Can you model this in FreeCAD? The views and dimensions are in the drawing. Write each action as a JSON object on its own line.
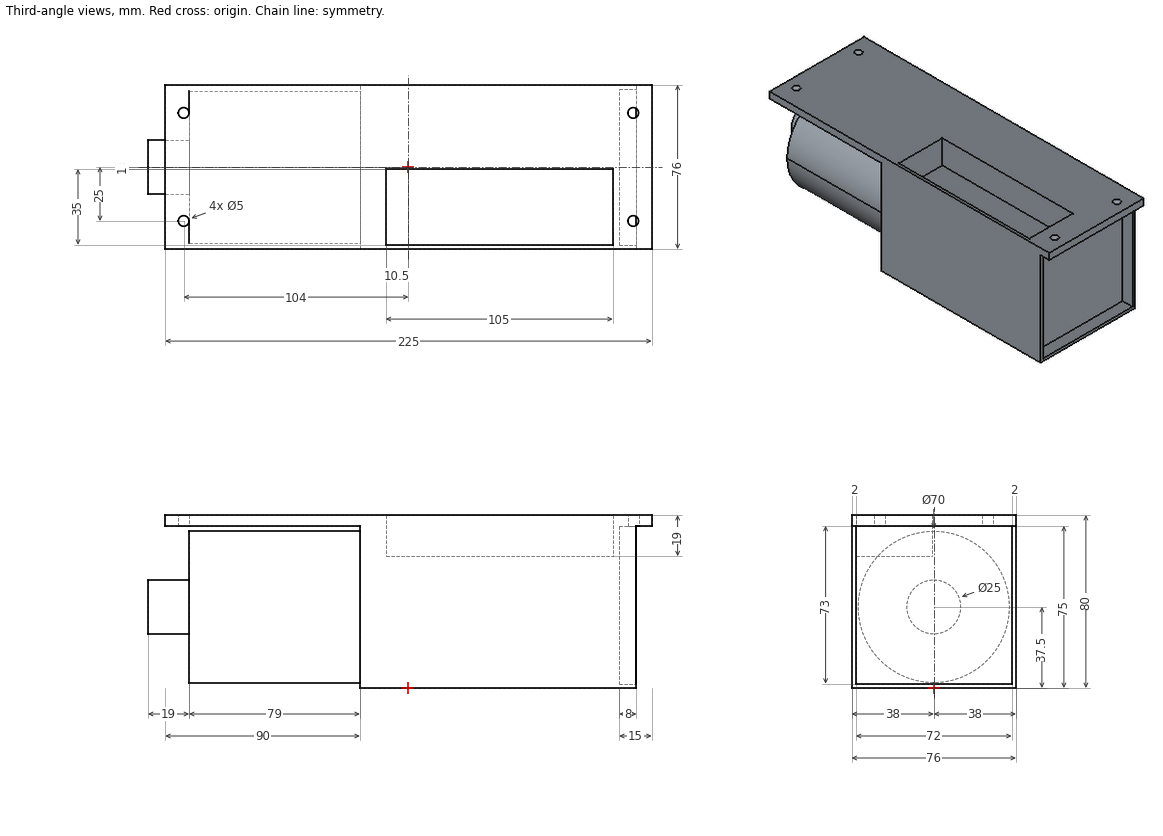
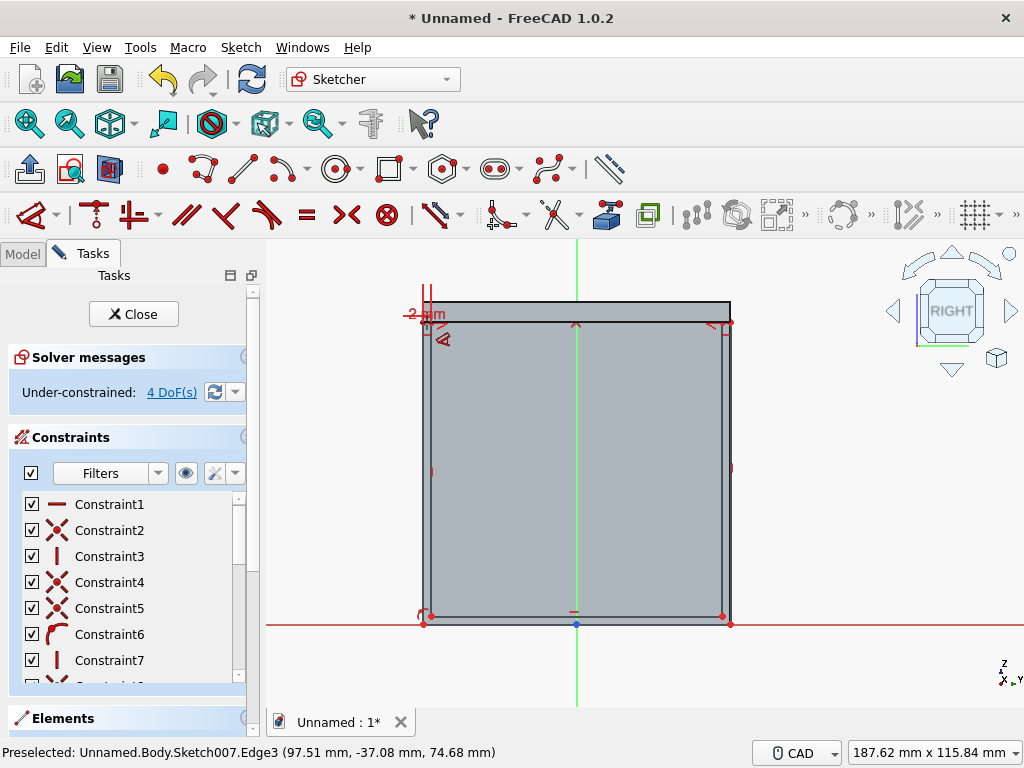
{"action": "scroll", "coordinate": [728, 323], "scroll_direction": "up", "scroll_amount": 9}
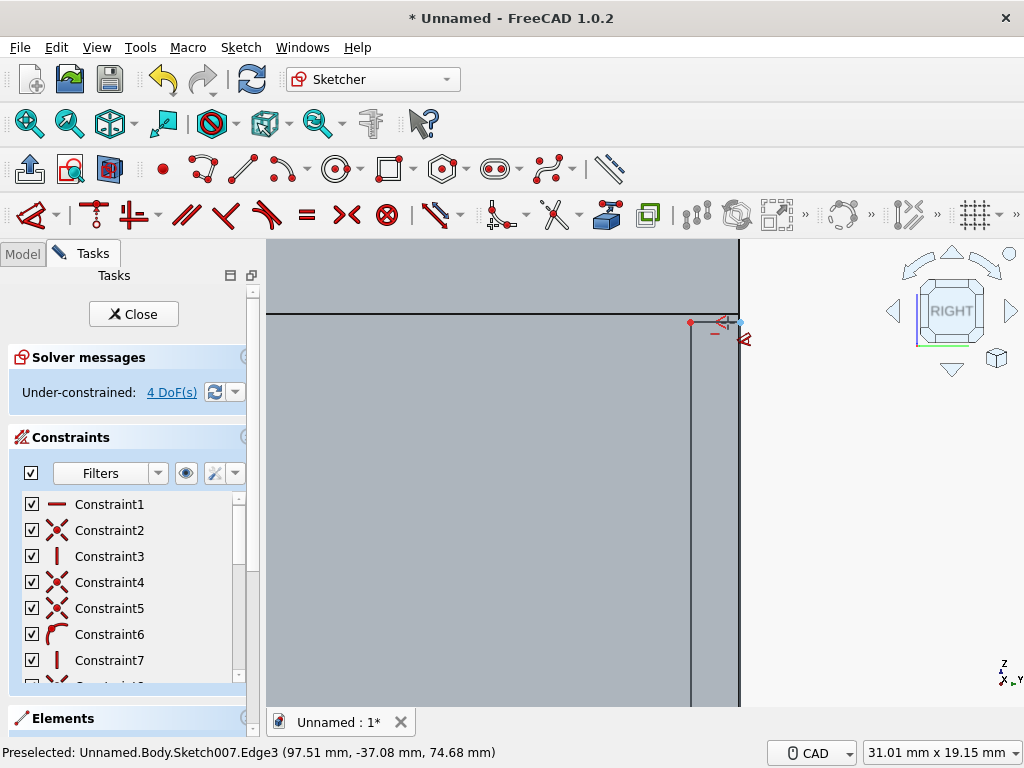
{"action": "left_click", "coordinate": [725, 322]}
{"action": "left_click", "coordinate": [715, 288]}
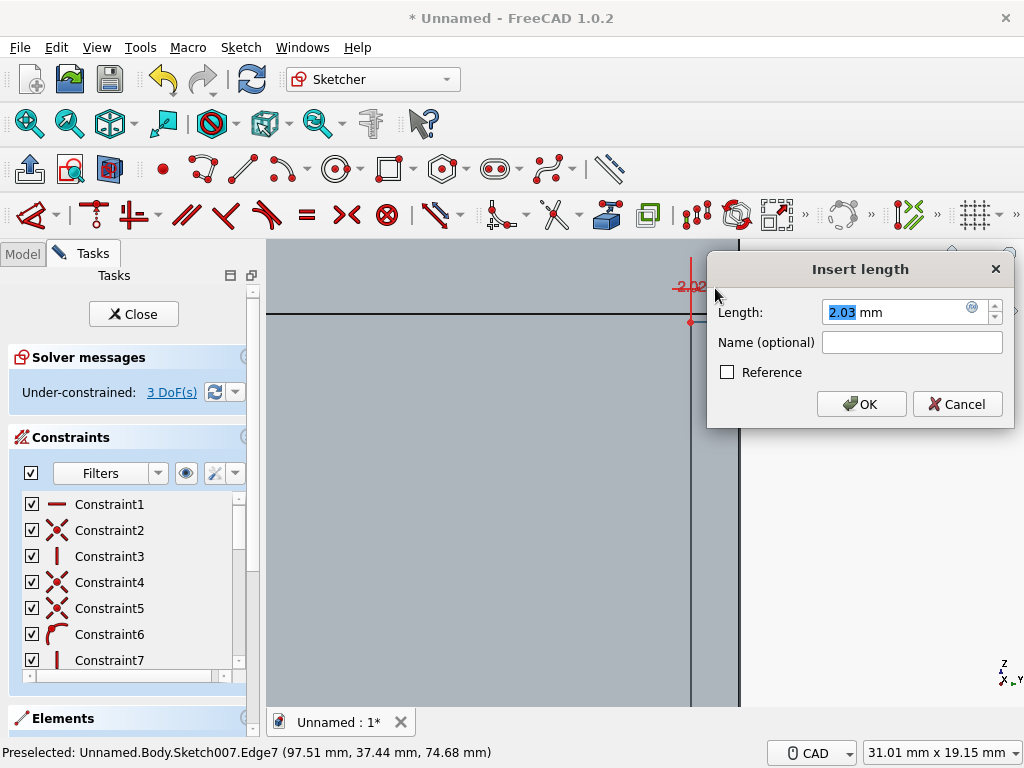
{"action": "type", "text": "2"}
{"action": "key", "text": "Return"}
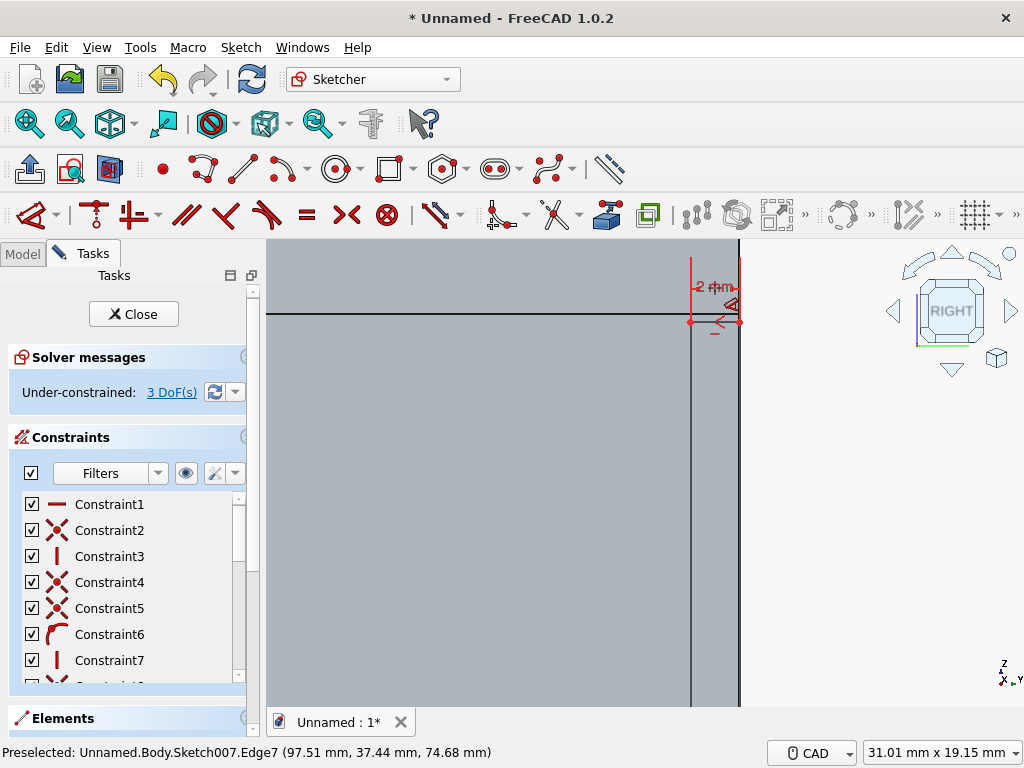
{"action": "scroll", "coordinate": [728, 323], "scroll_direction": "down", "scroll_amount": 9}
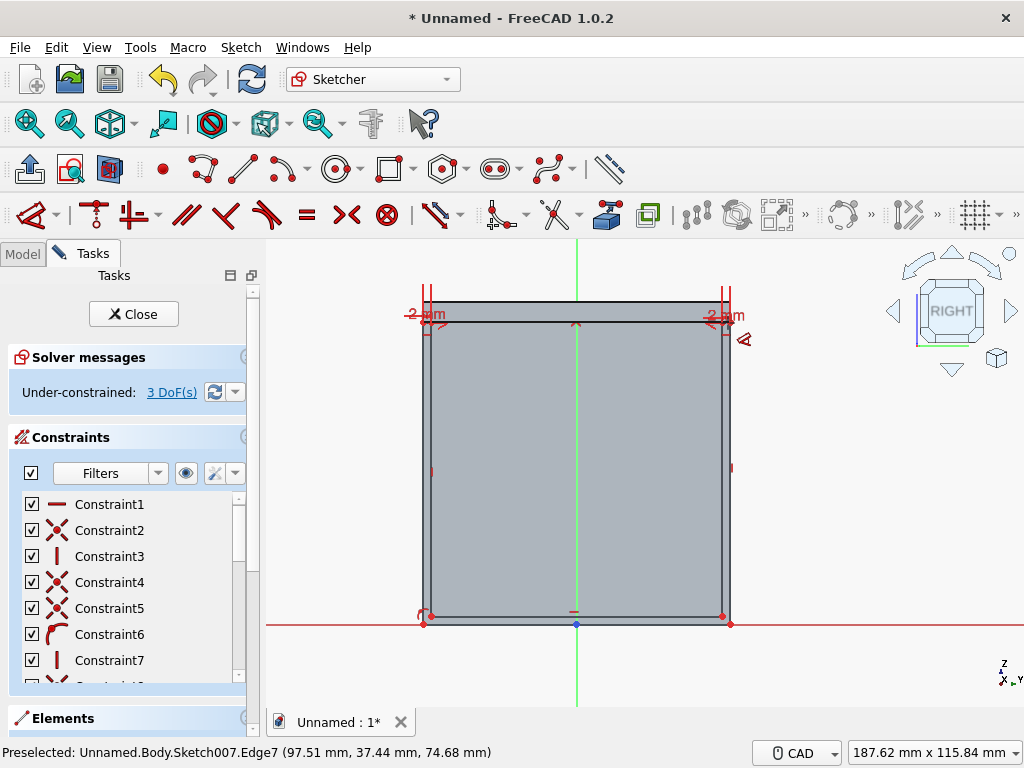
{"action": "scroll", "coordinate": [635, 617], "scroll_direction": "up", "scroll_amount": 3}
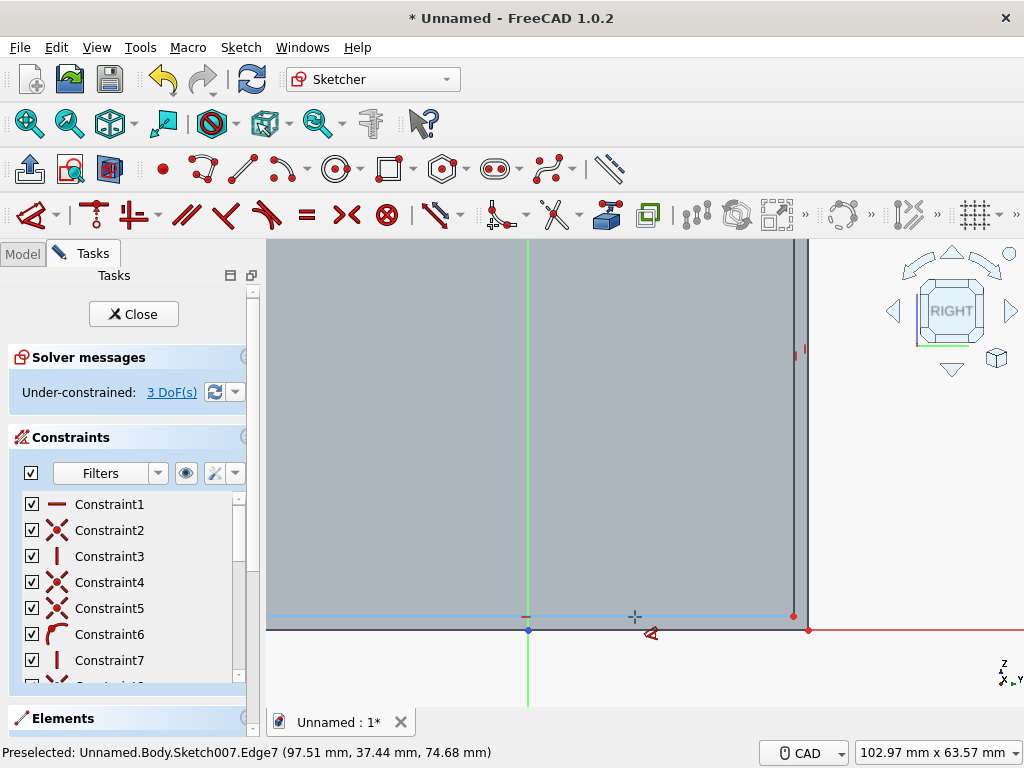
{"action": "left_click", "coordinate": [635, 616]}
{"action": "left_click", "coordinate": [544, 650]}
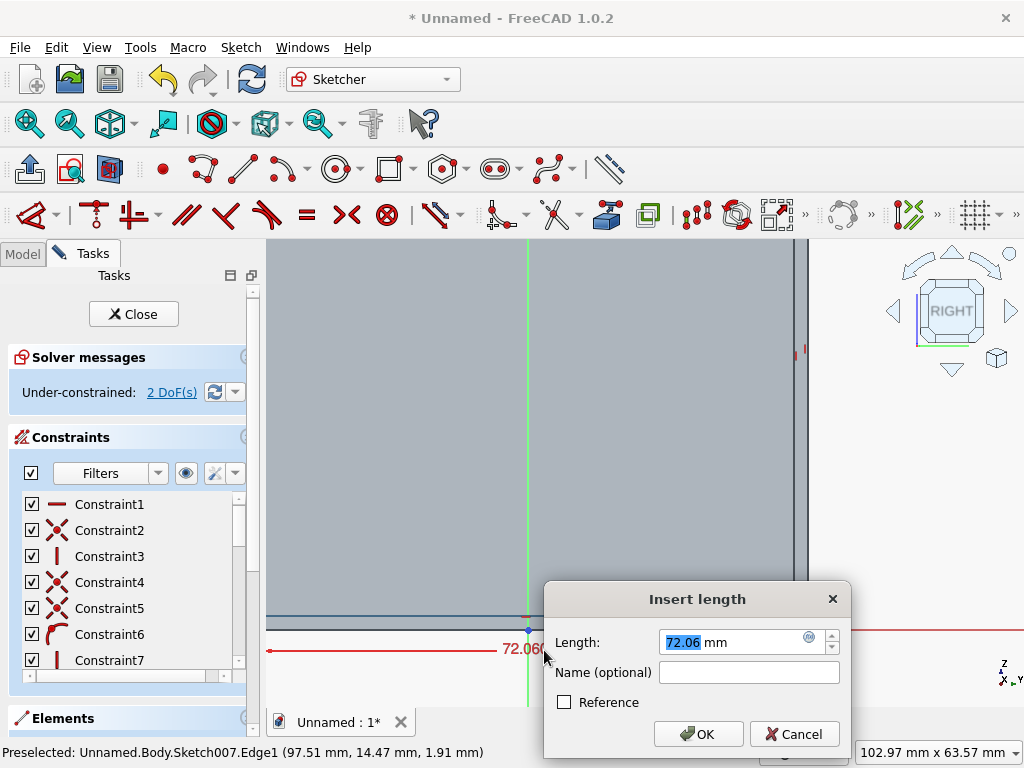
{"action": "type", "text": "72"}
{"action": "key", "text": "Return"}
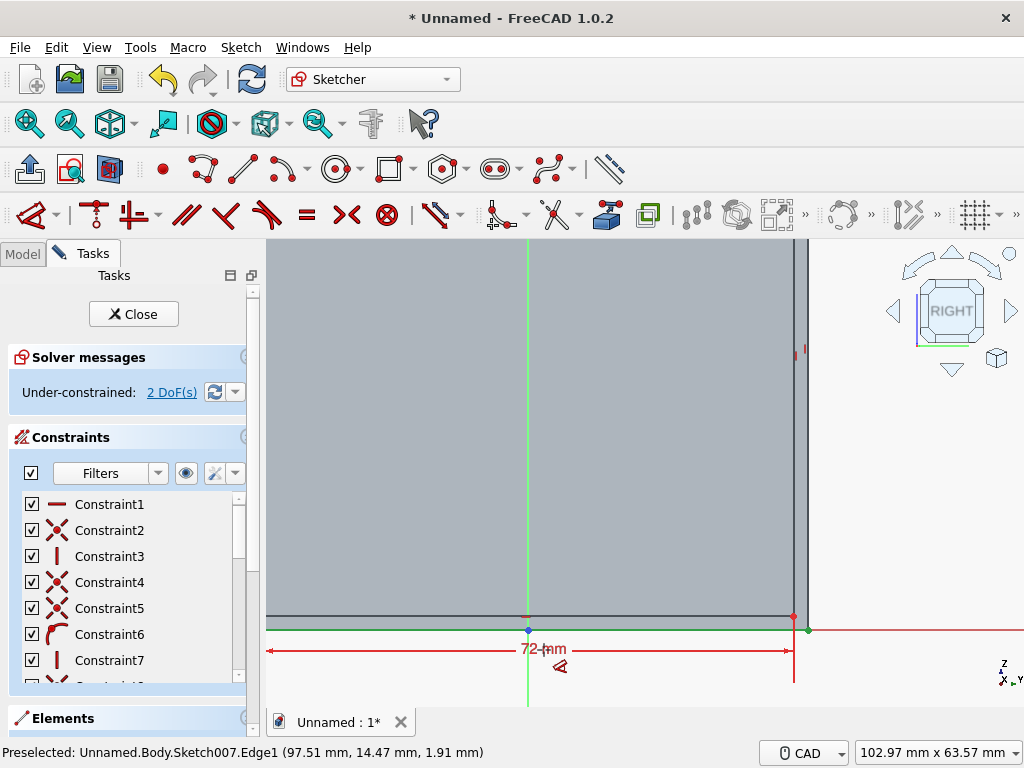
{"action": "scroll", "coordinate": [635, 617], "scroll_direction": "down", "scroll_amount": 3}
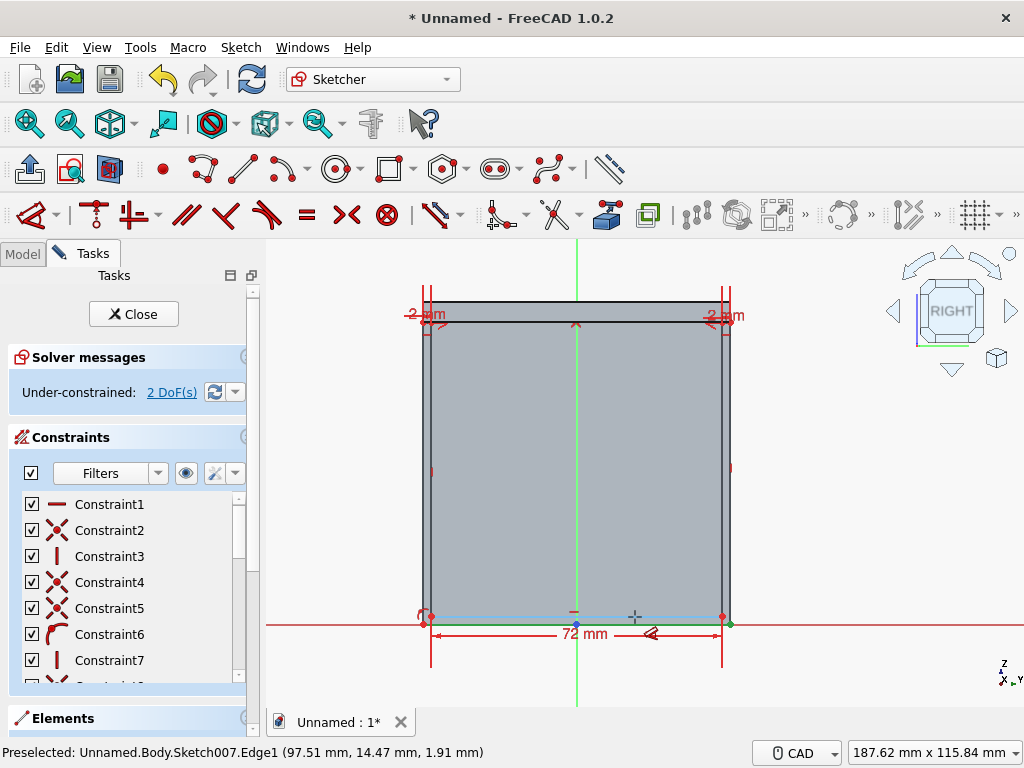
{"action": "scroll", "coordinate": [431, 529], "scroll_direction": "up", "scroll_amount": 3}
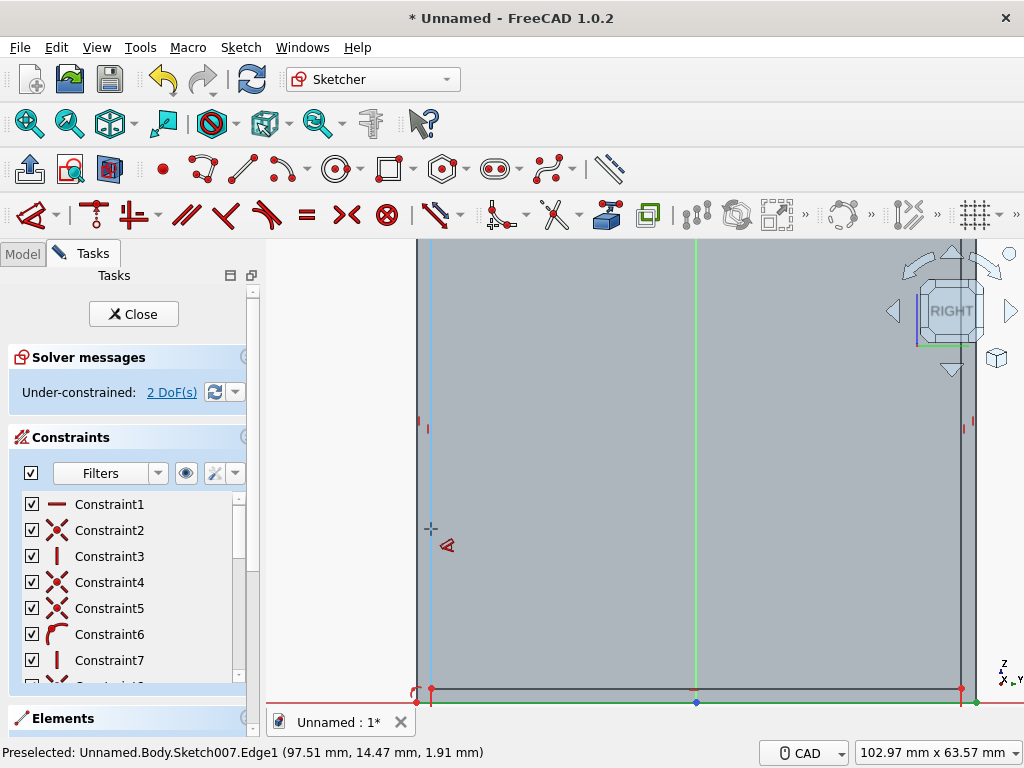
{"action": "left_click", "coordinate": [431, 528]}
{"action": "left_click", "coordinate": [397, 473]}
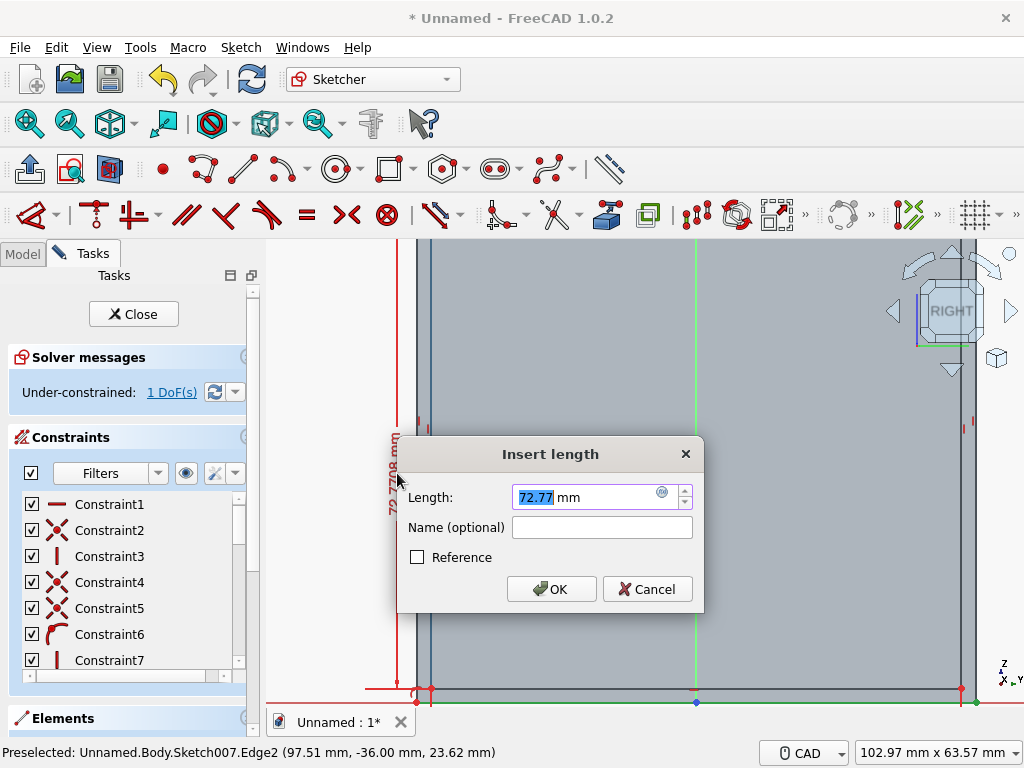
{"action": "type", "text": "73"}
{"action": "key", "text": "Return"}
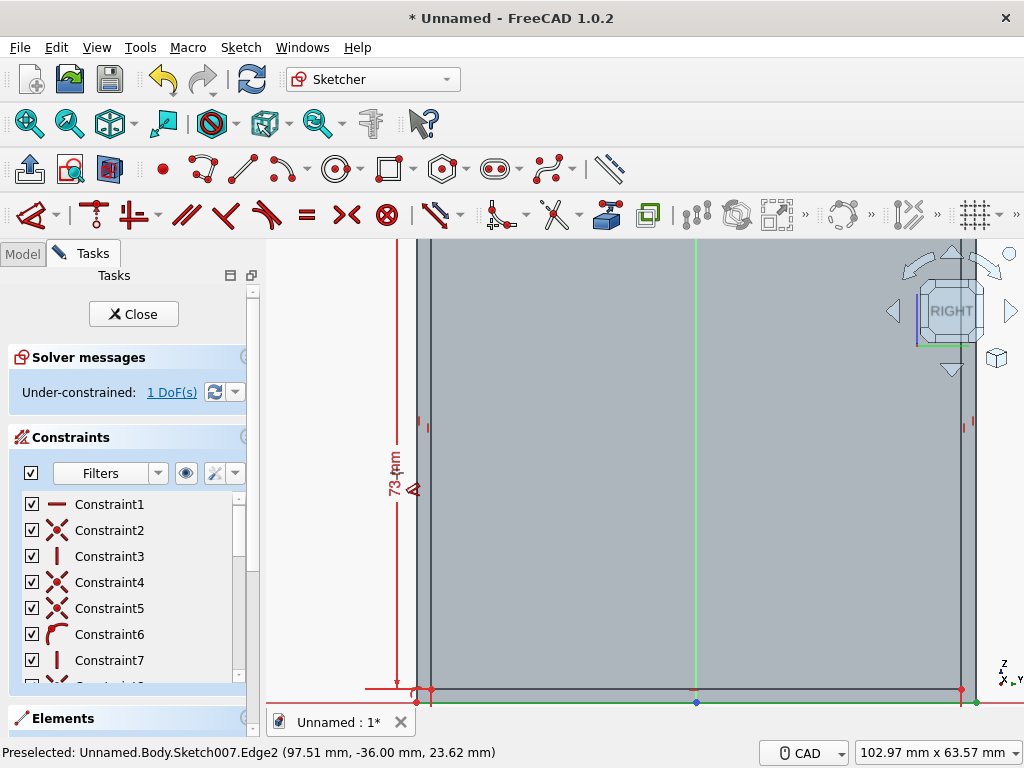
{"action": "left_click", "coordinate": [417, 317]}
{"action": "left_click", "coordinate": [383, 378]}